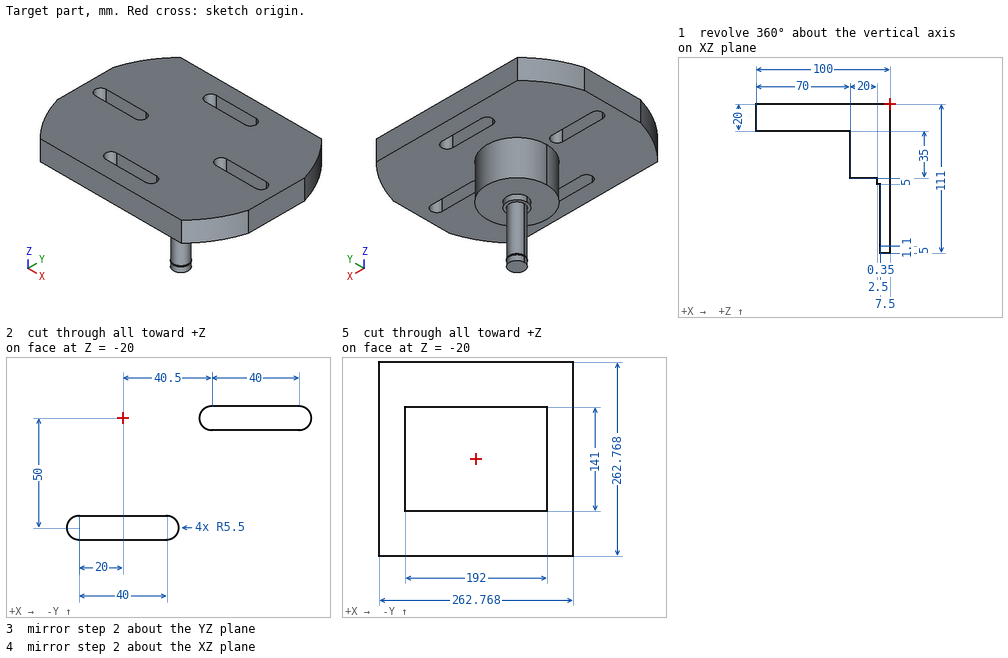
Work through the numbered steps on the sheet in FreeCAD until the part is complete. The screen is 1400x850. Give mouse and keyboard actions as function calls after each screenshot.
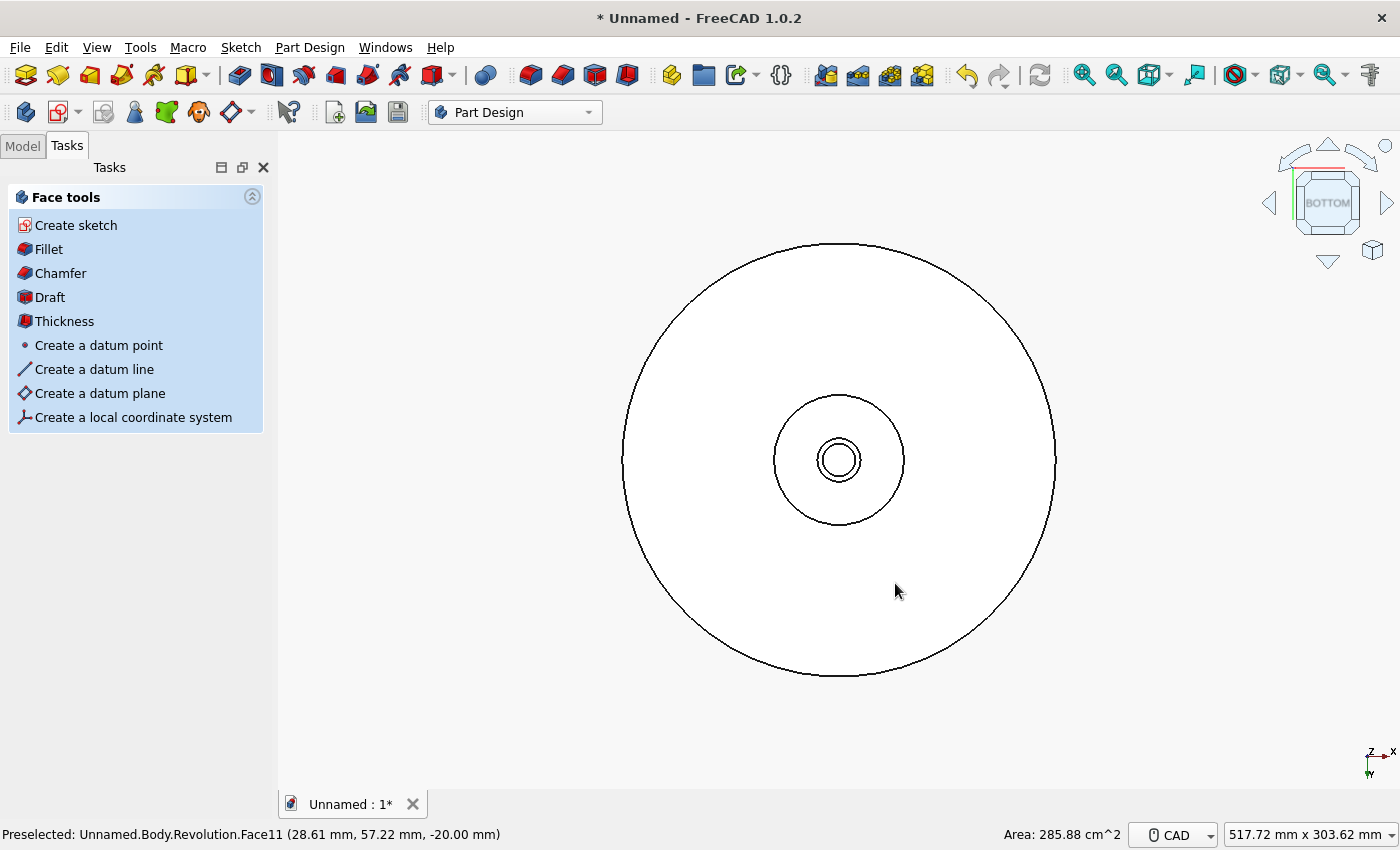
click(58, 112)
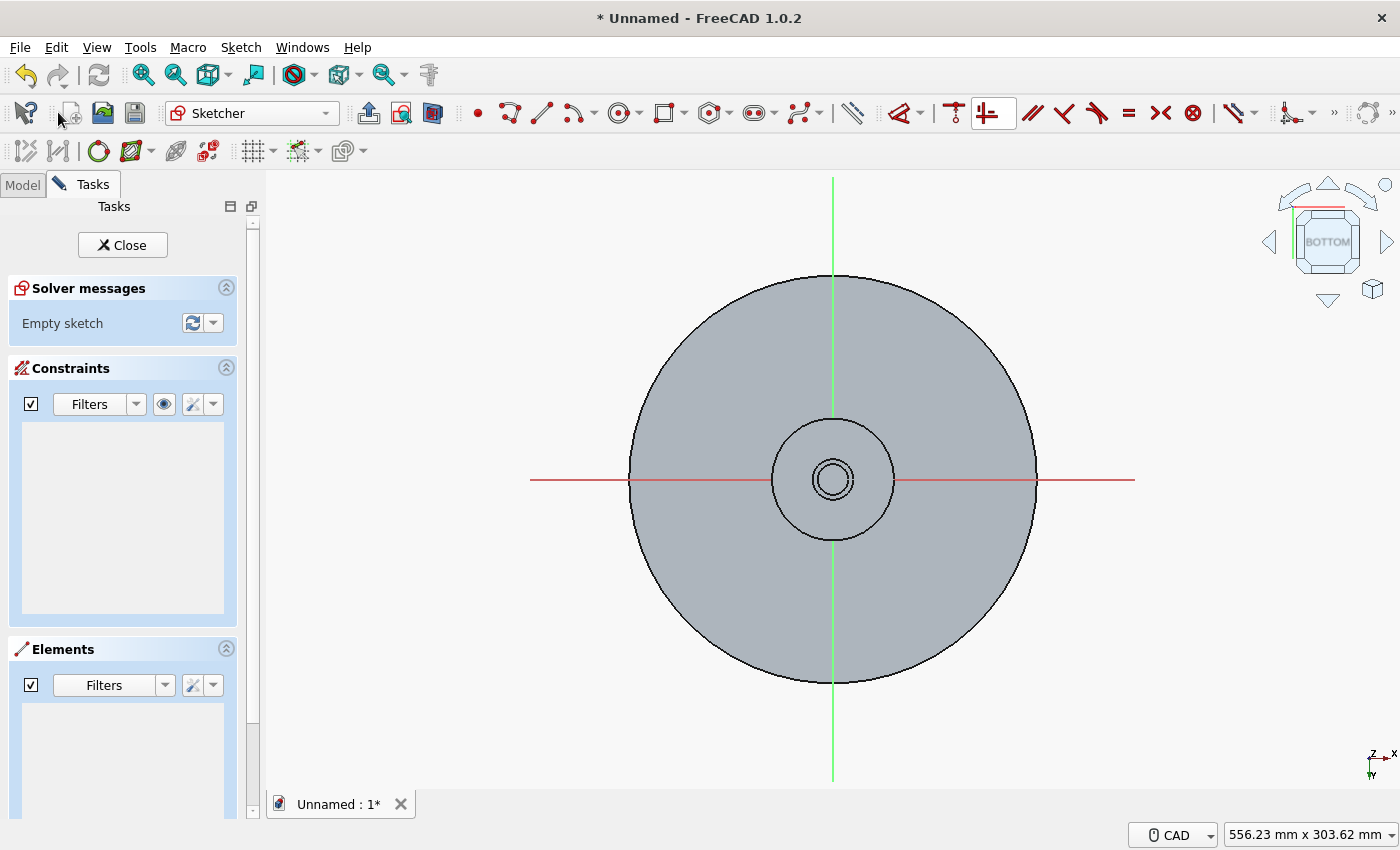
scroll(970, 560, up, 5)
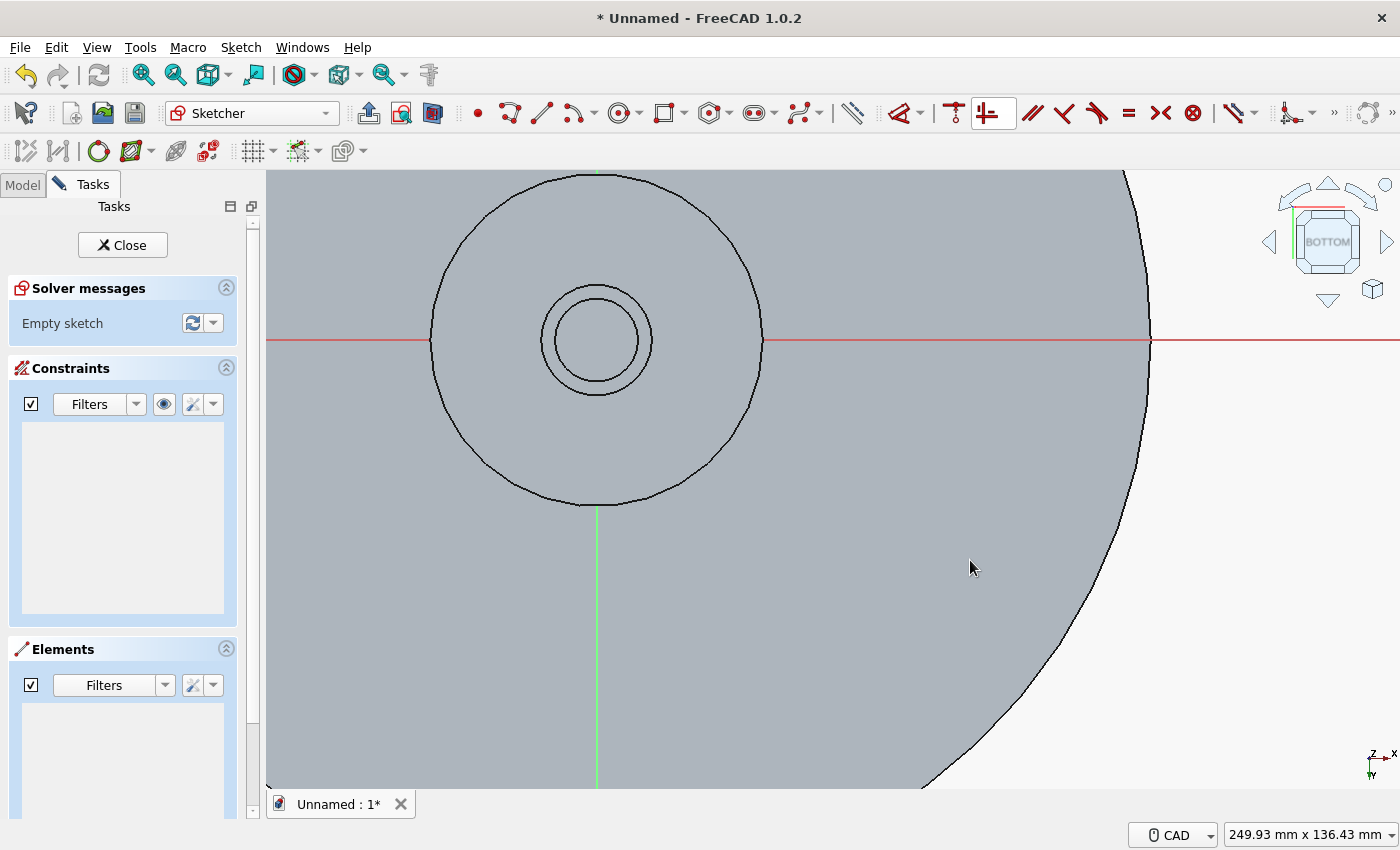
key(g)
key(s)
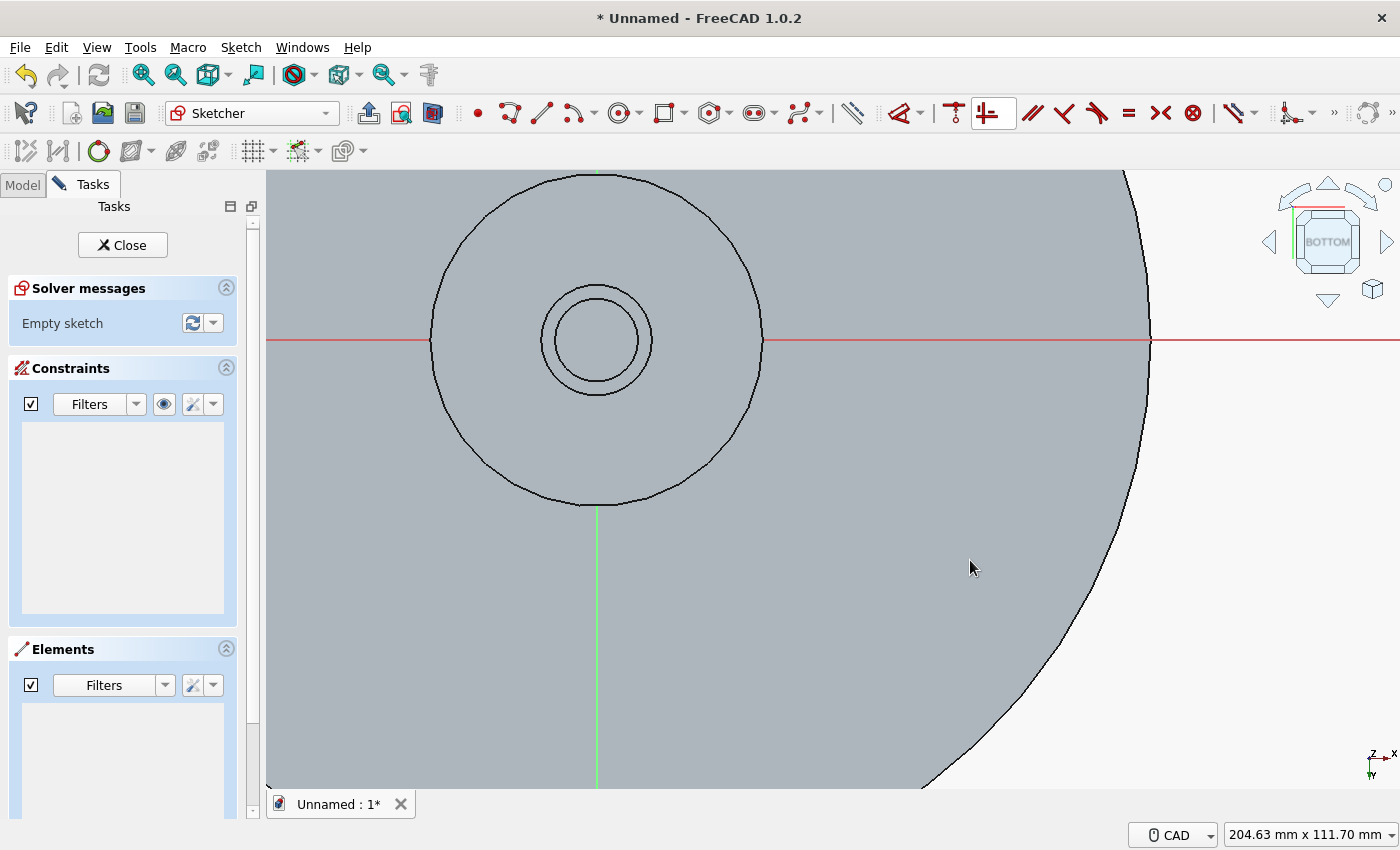
click(486, 617)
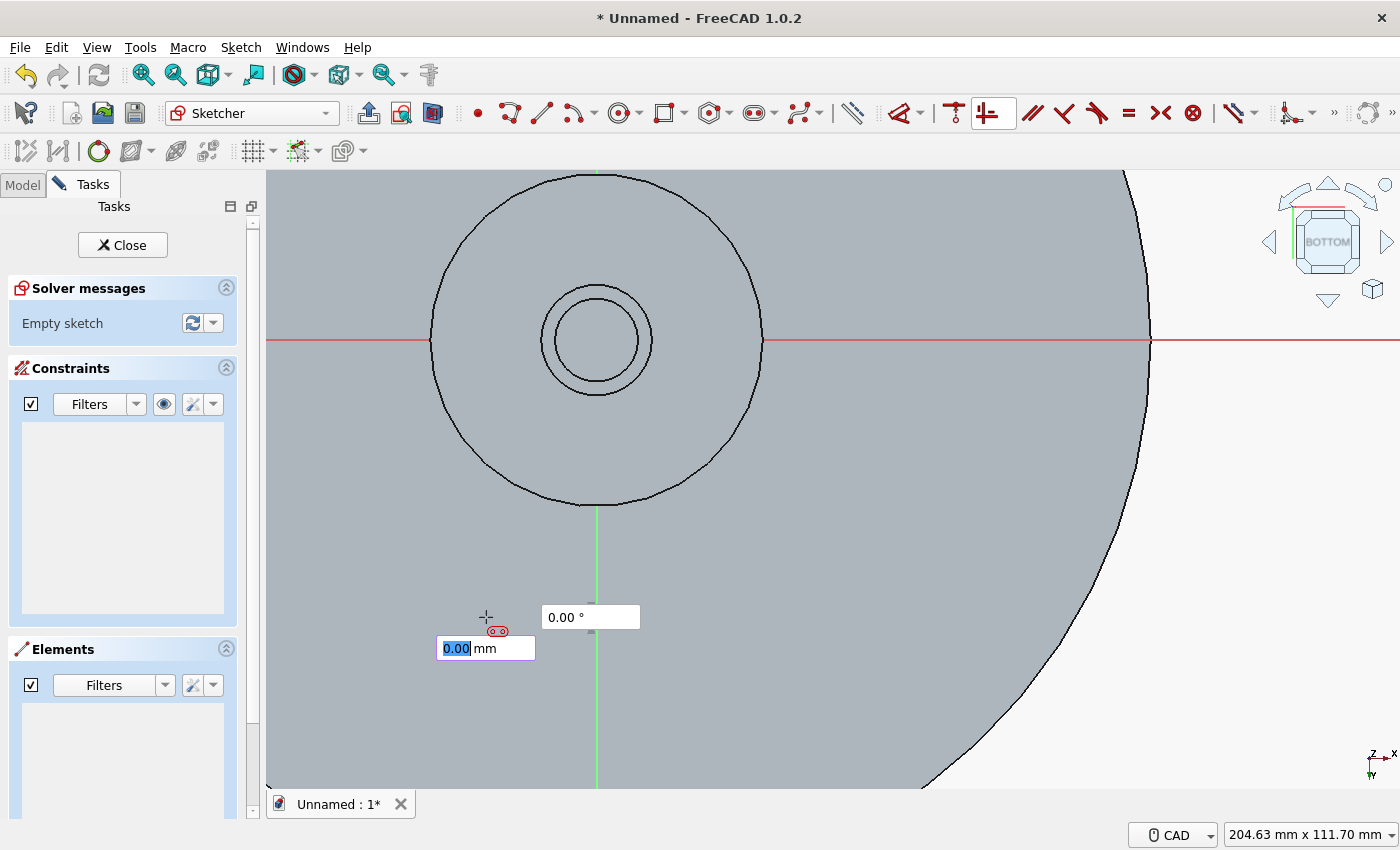
click(707, 617)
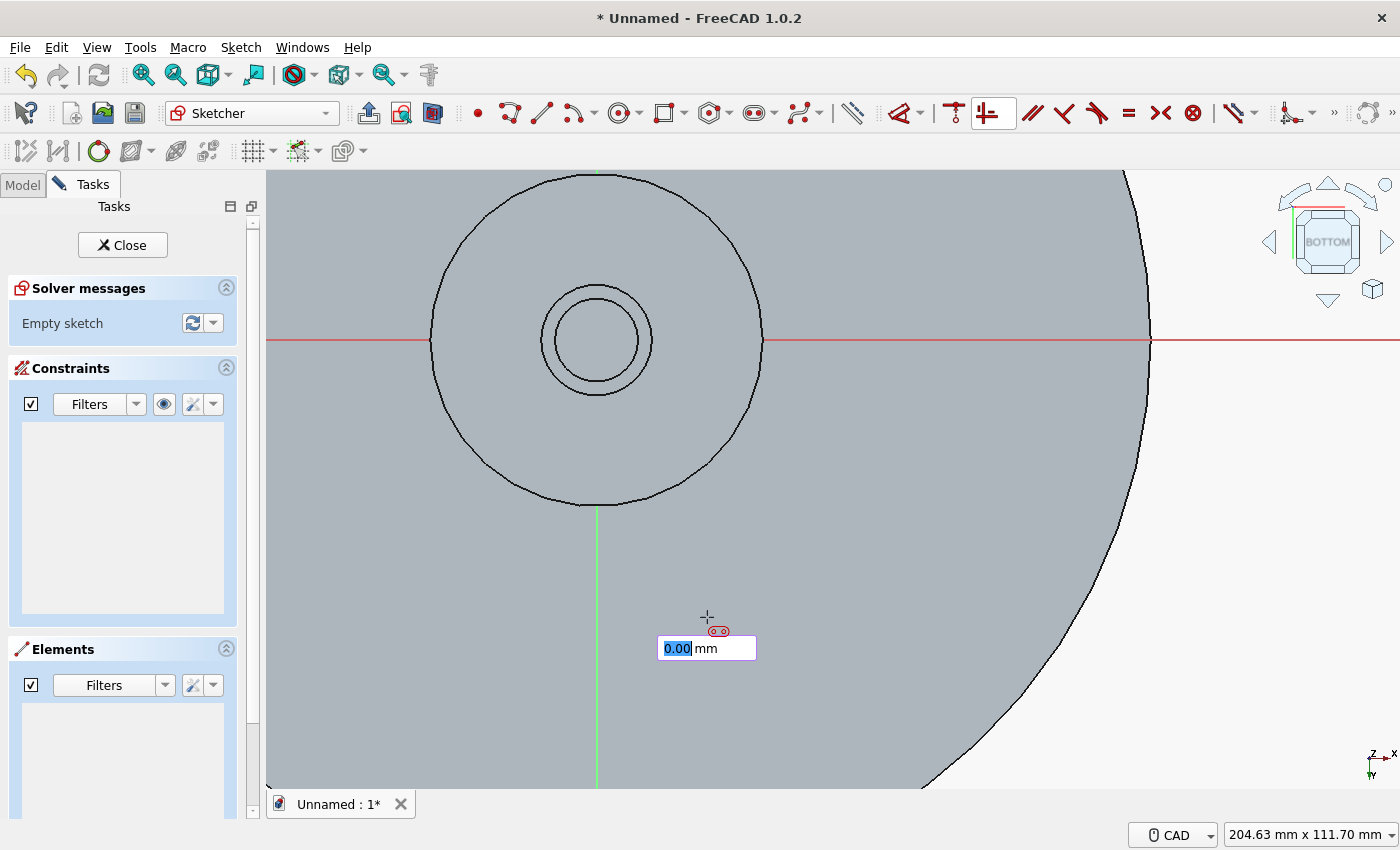
click(563, 648)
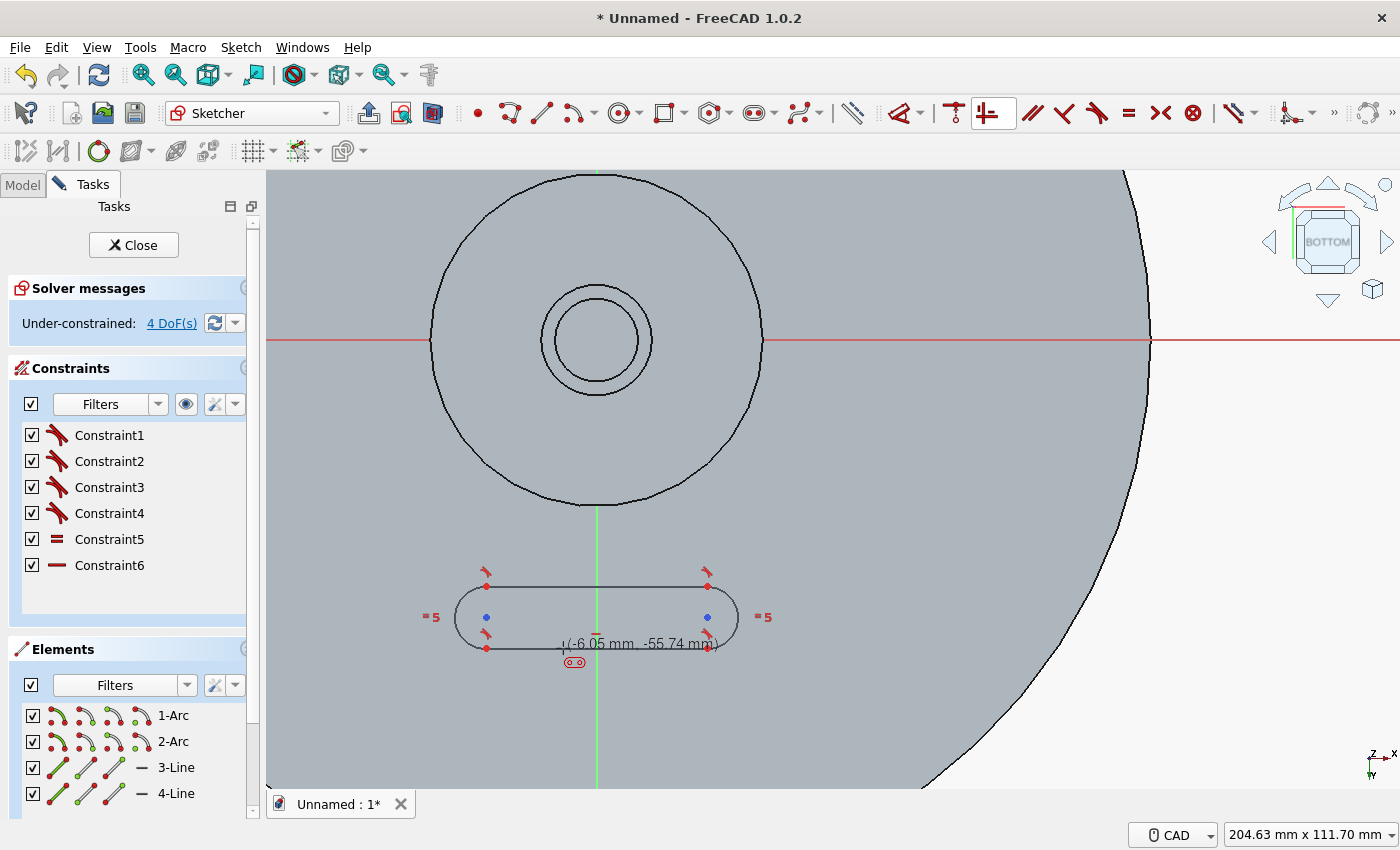
click(821, 340)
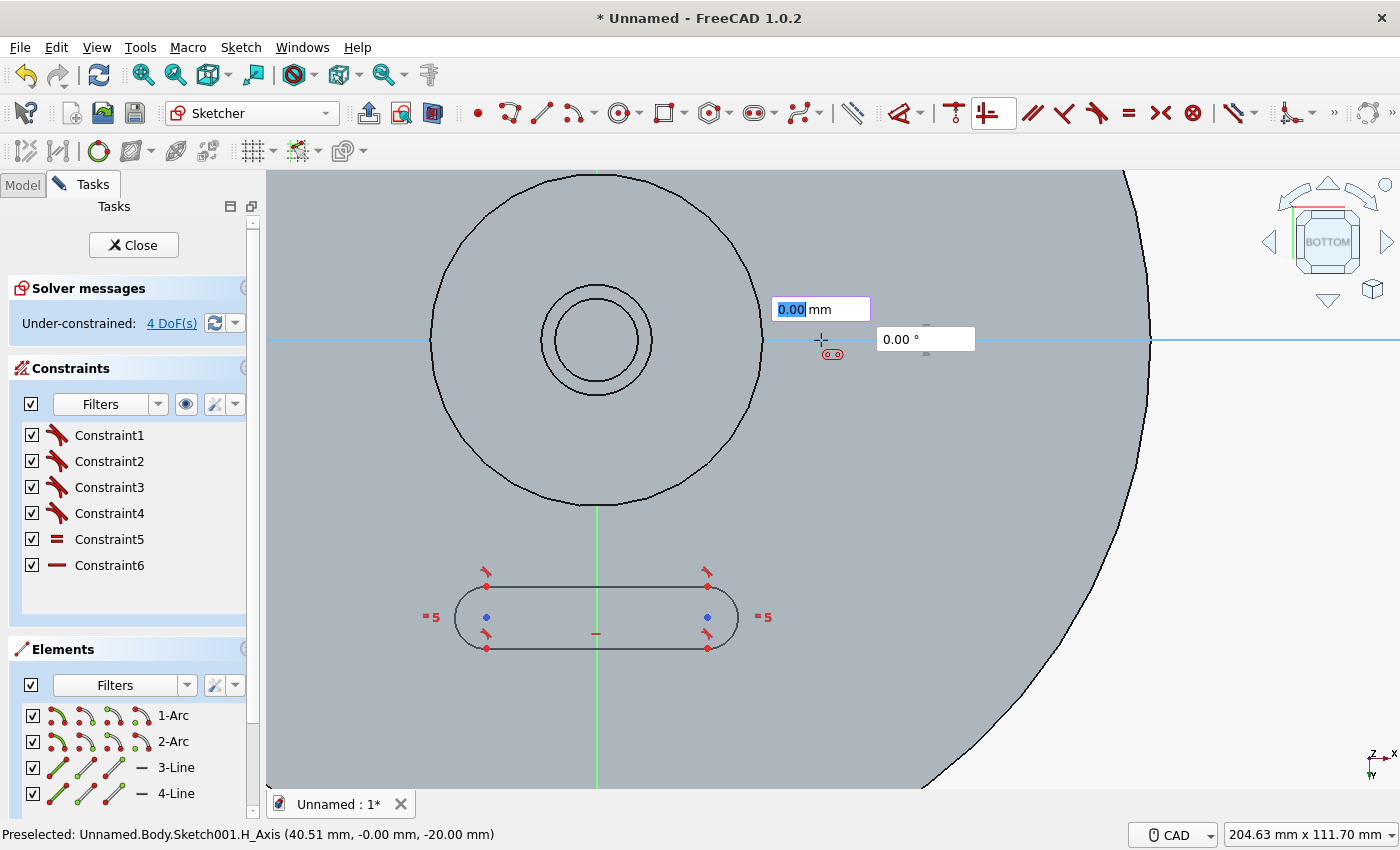
click(1043, 349)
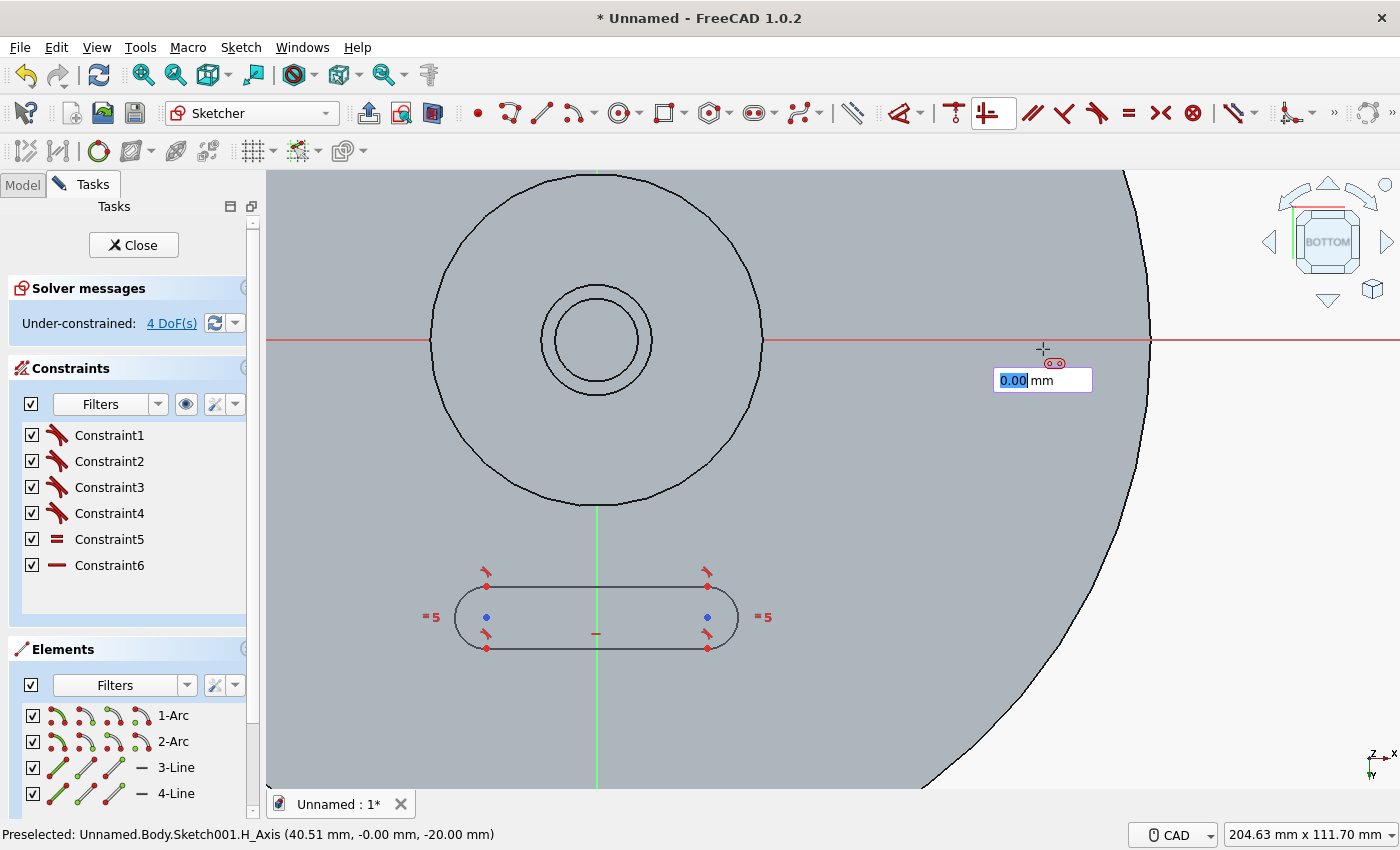
click(932, 310)
key(Escape)